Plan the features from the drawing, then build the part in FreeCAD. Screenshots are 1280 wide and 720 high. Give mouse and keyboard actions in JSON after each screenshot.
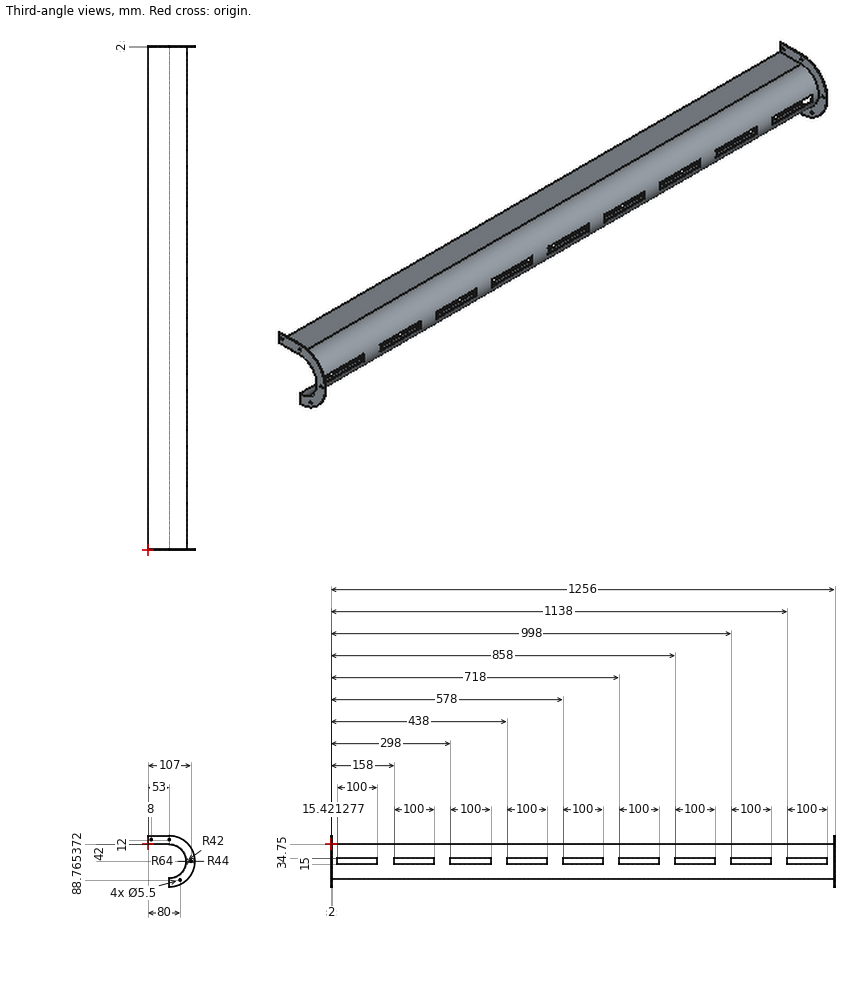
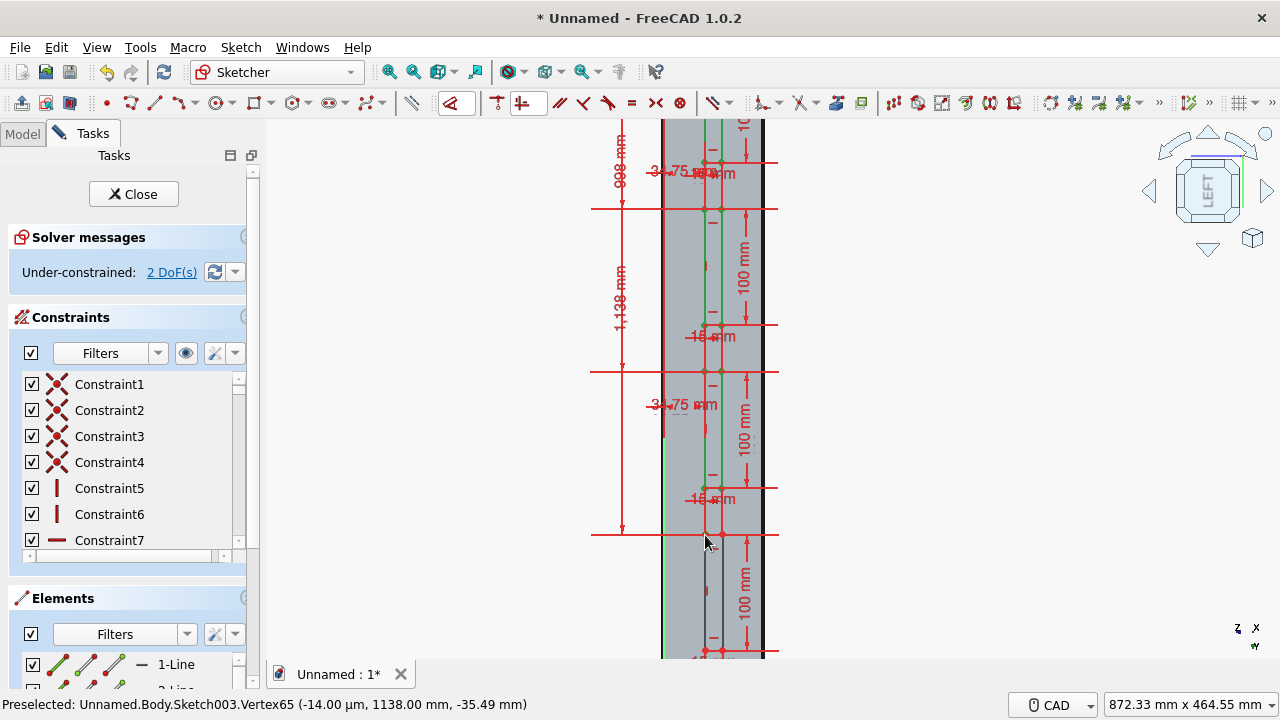
{"action": "key", "text": "l"}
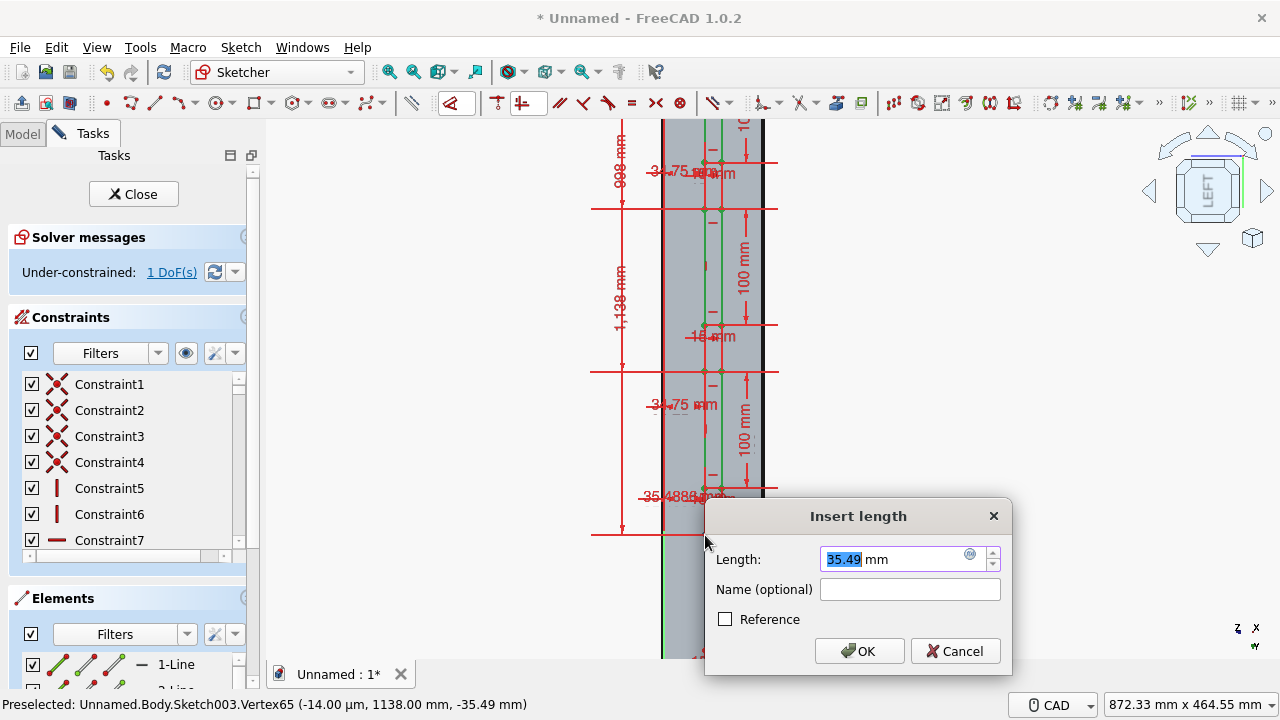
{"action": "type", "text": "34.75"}
{"action": "key", "text": "Return"}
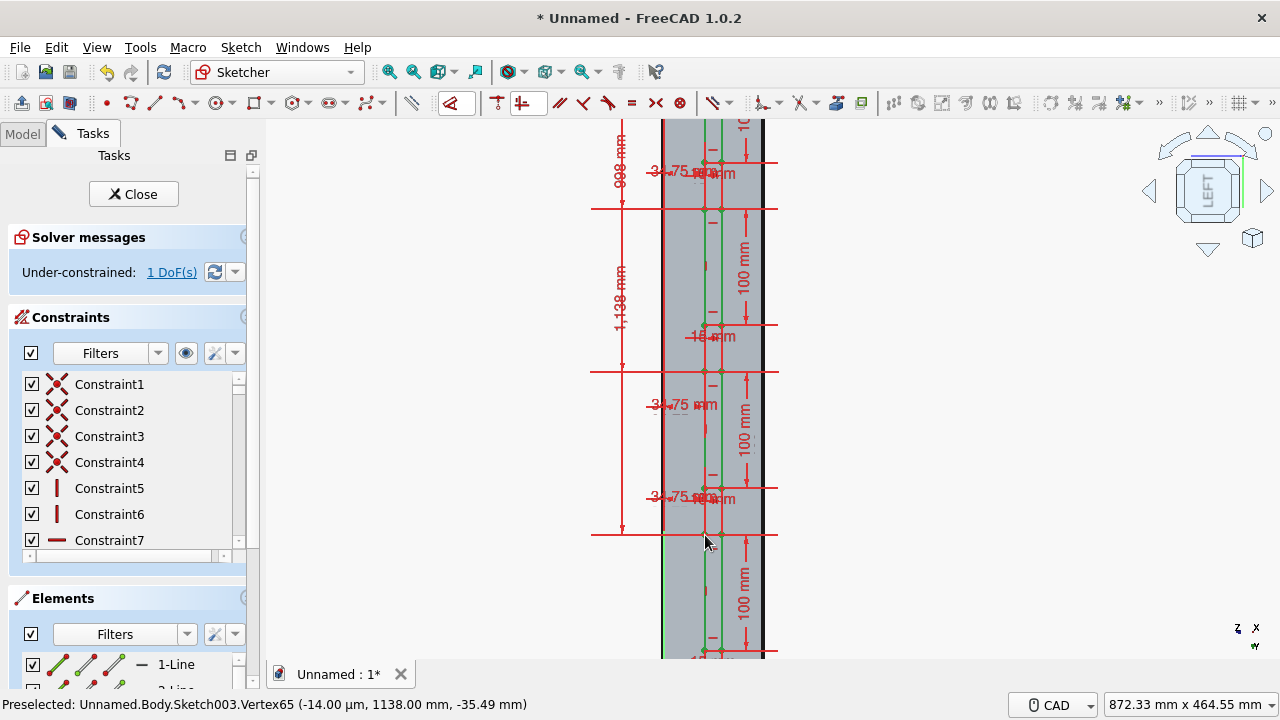
{"action": "scroll", "coordinate": [708, 539], "scroll_direction": "down", "scroll_amount": 7}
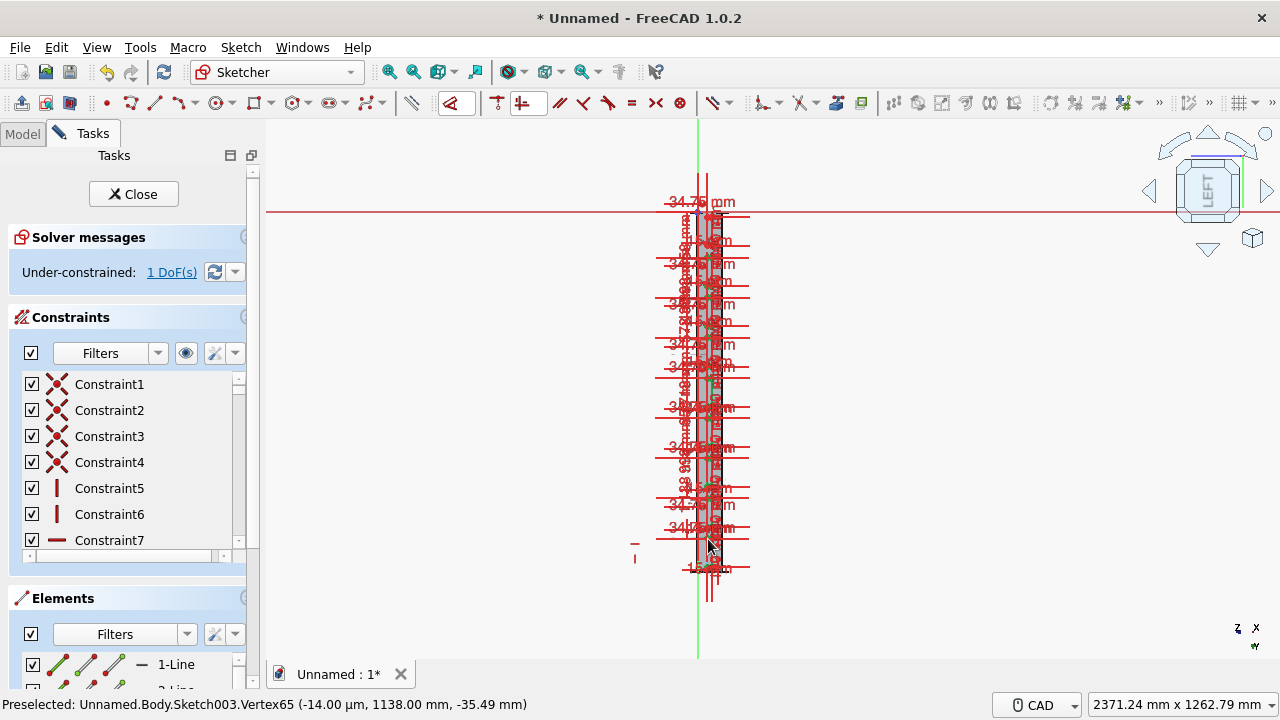
{"action": "scroll", "coordinate": [707, 217], "scroll_direction": "up", "scroll_amount": 11}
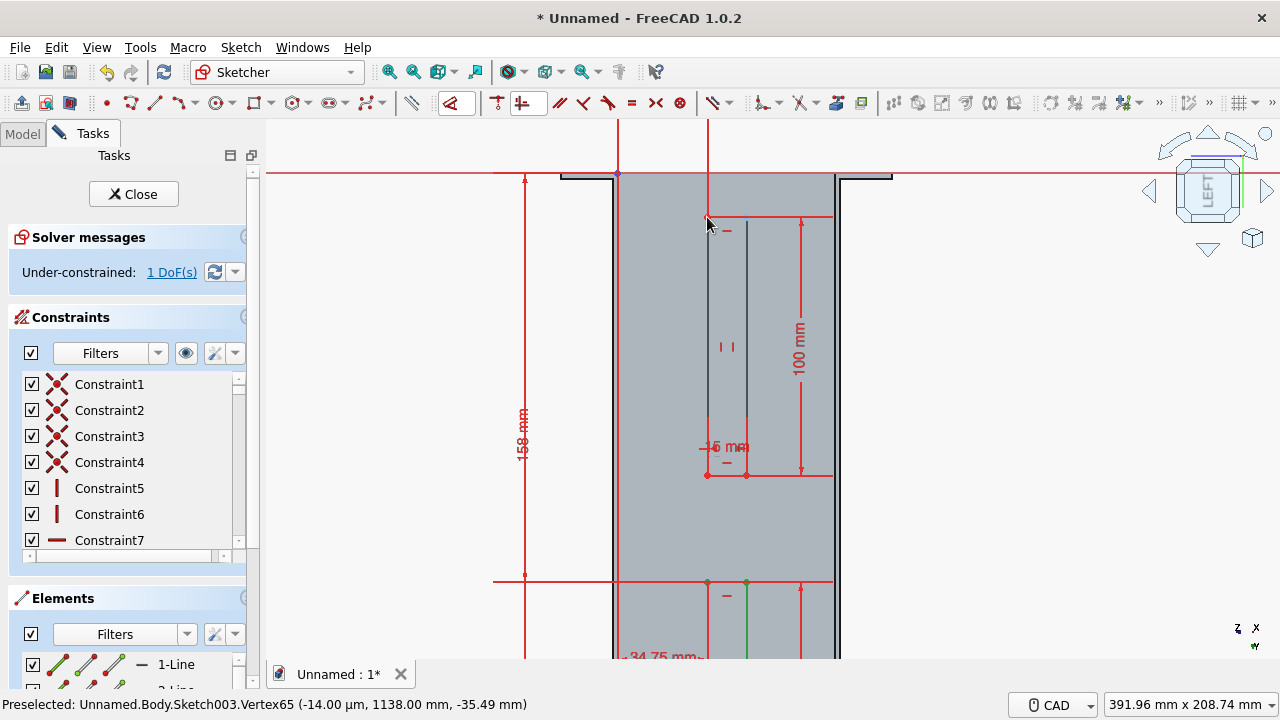
{"action": "left_click", "coordinate": [708, 217]}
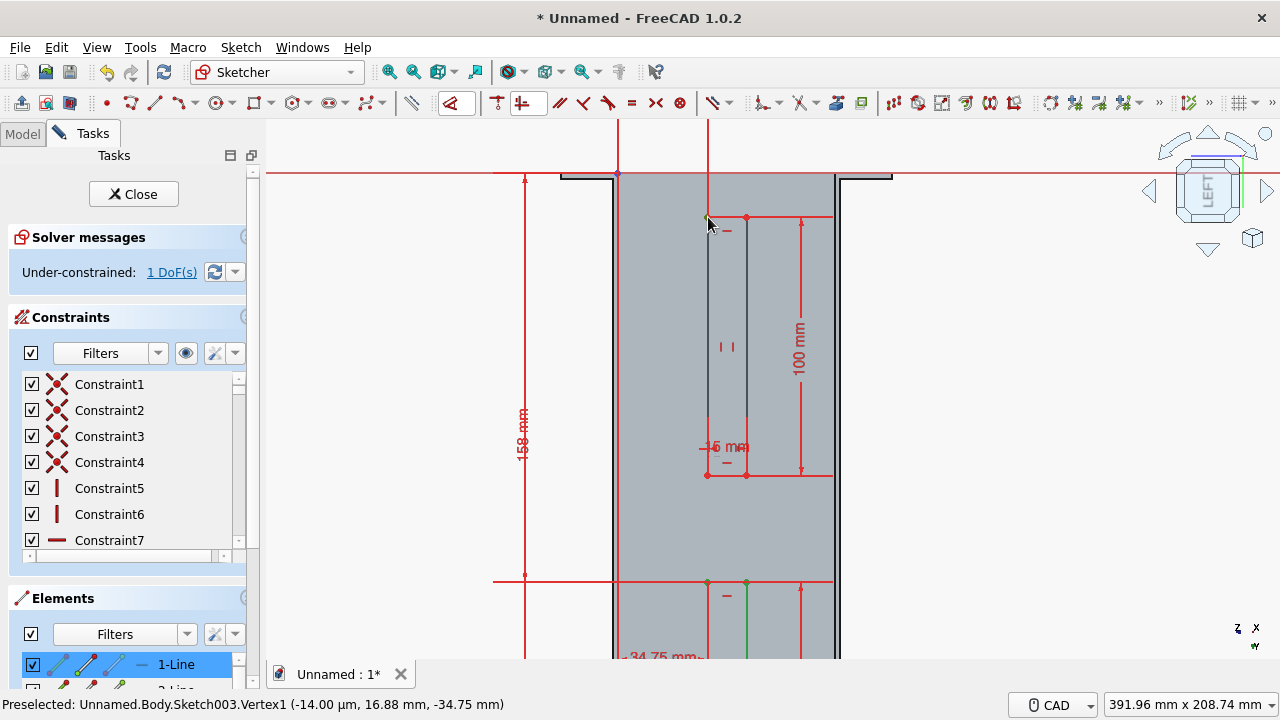
{"action": "left_click", "coordinate": [470, 104]}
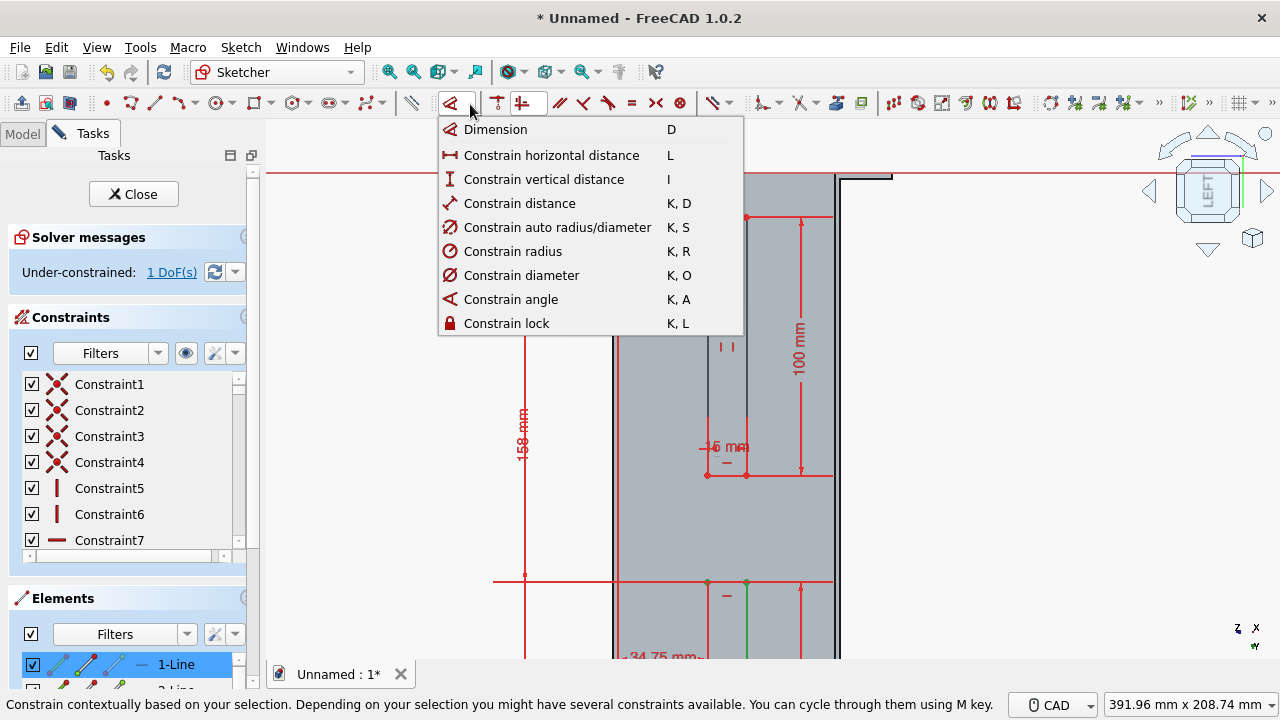
{"action": "left_click", "coordinate": [591, 179]}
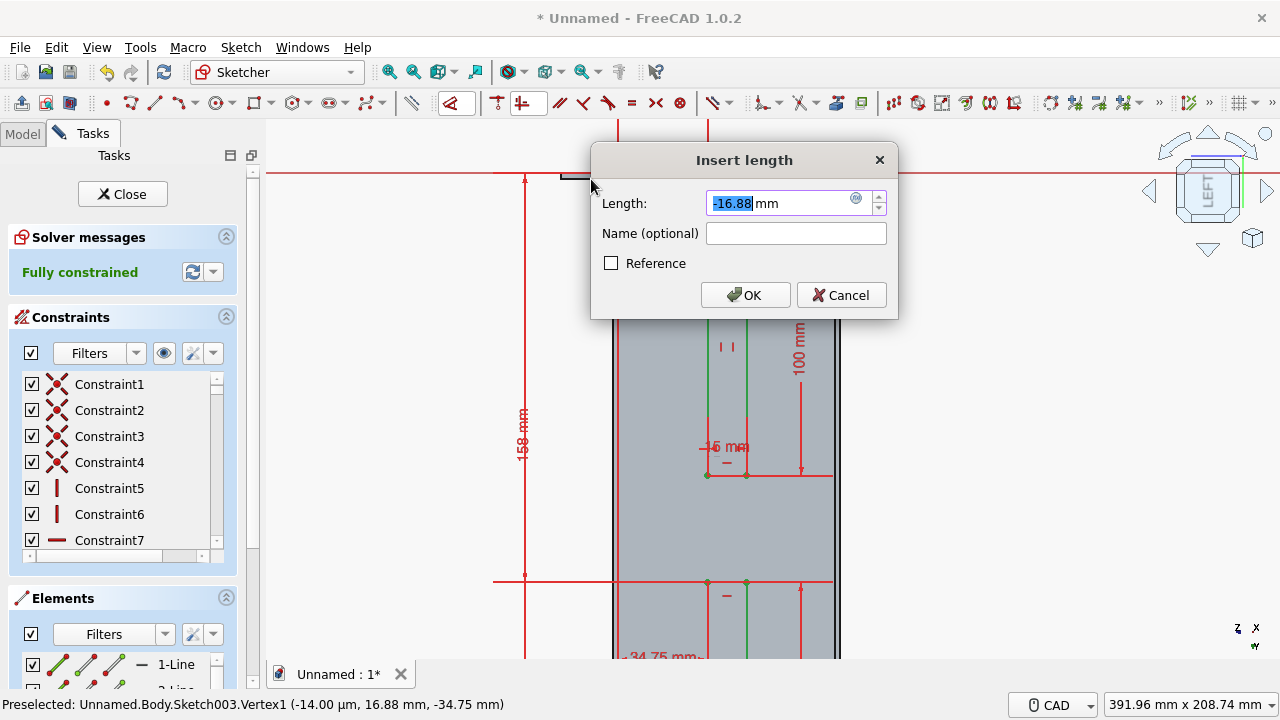
{"action": "type", "text": "-15.421277"}
{"action": "key", "text": "Return"}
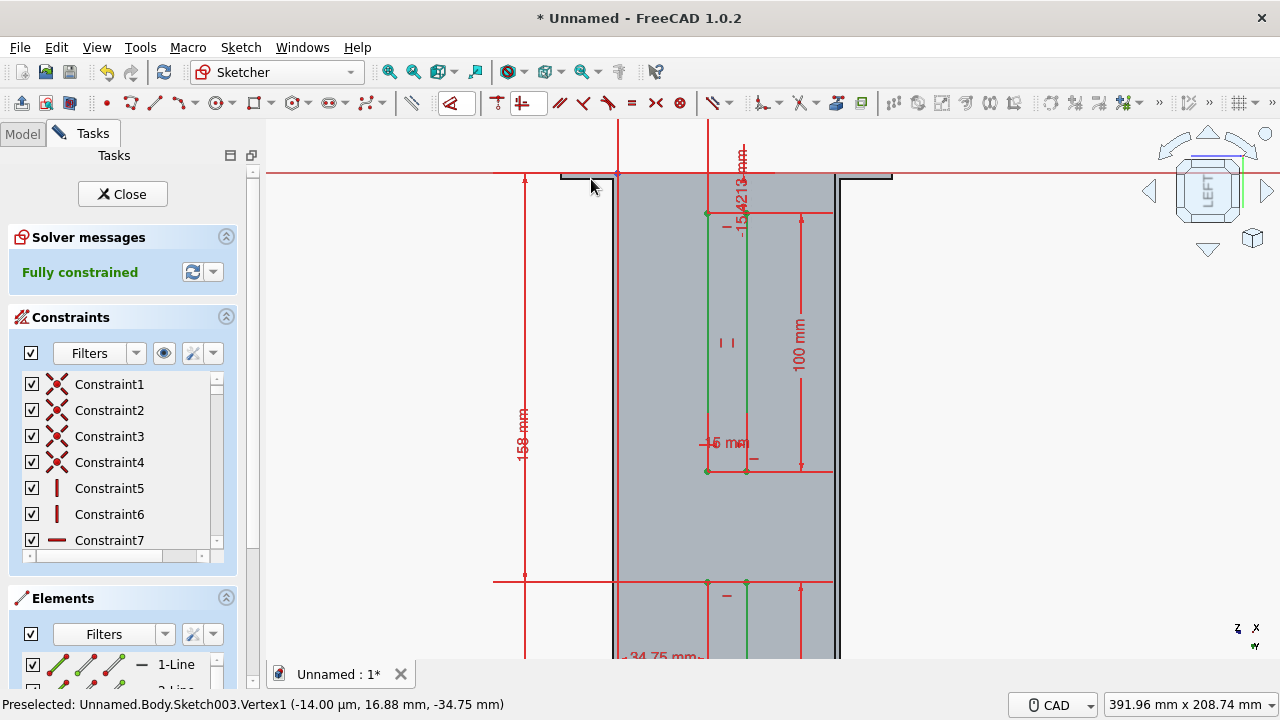
{"action": "left_click", "coordinate": [123, 194]}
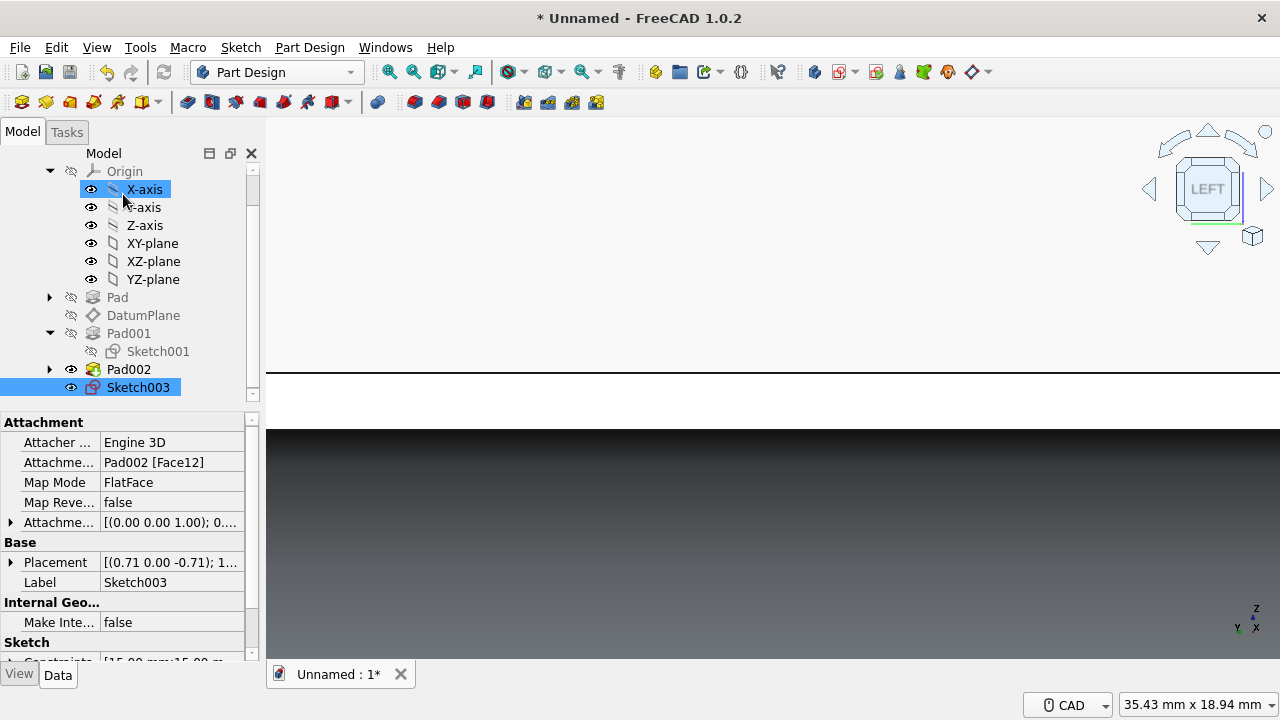
{"action": "left_click", "coordinate": [188, 102]}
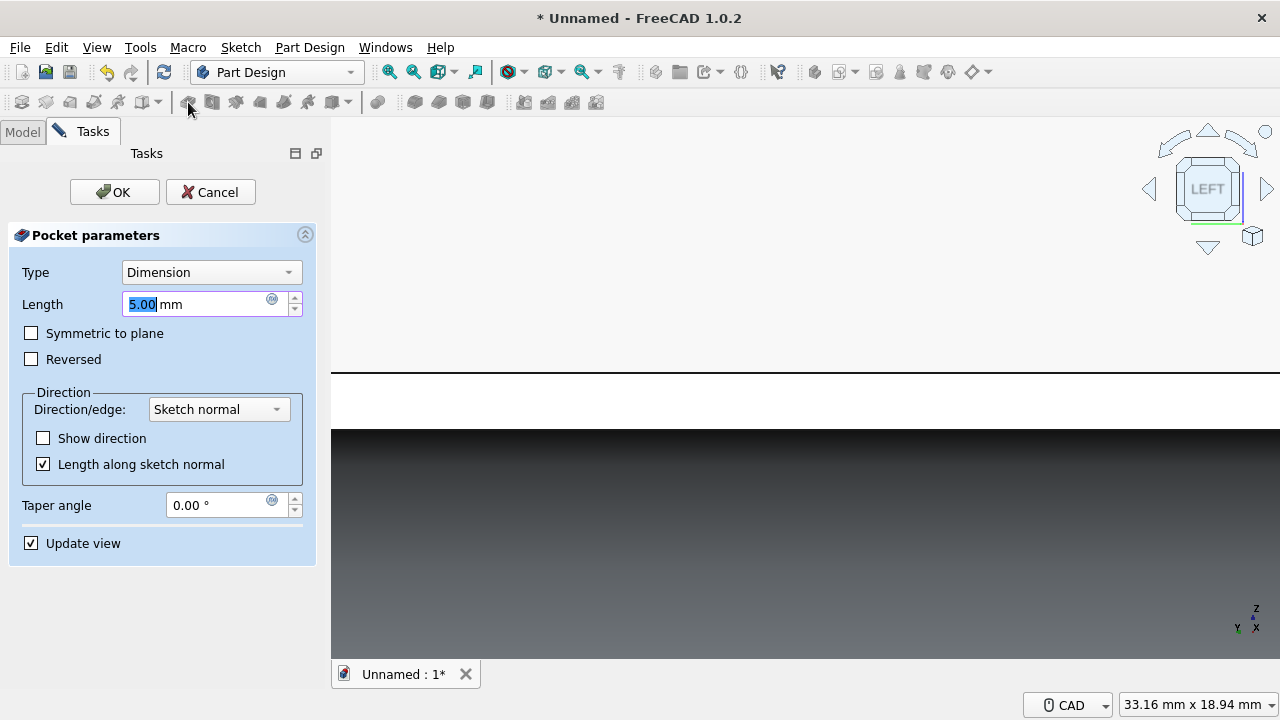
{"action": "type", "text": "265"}
{"action": "key", "text": "Tab"}